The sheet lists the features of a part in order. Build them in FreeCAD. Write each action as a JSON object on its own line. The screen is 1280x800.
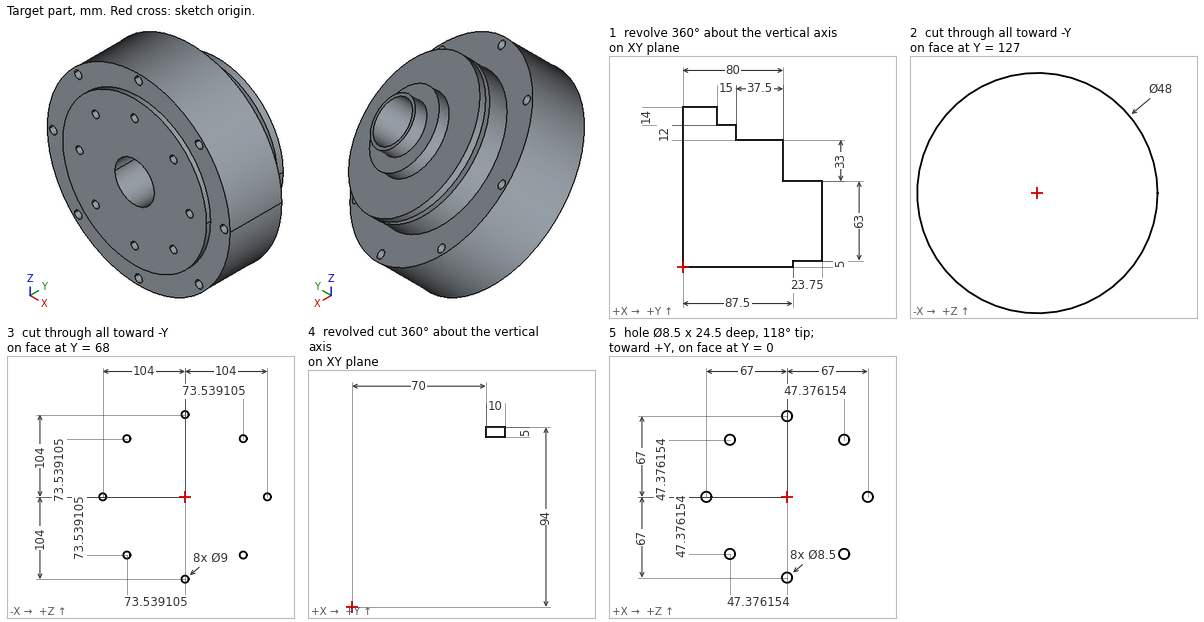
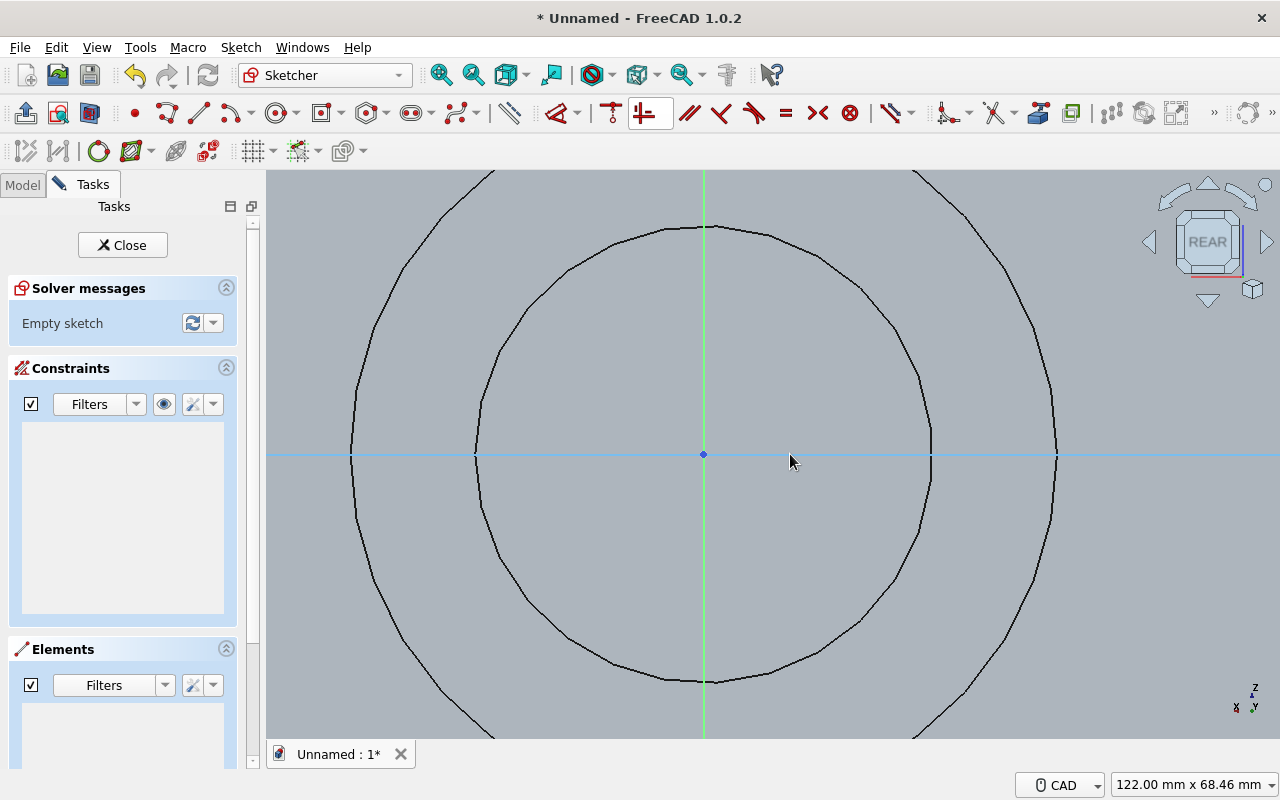
{"action": "left_click", "coordinate": [276, 114]}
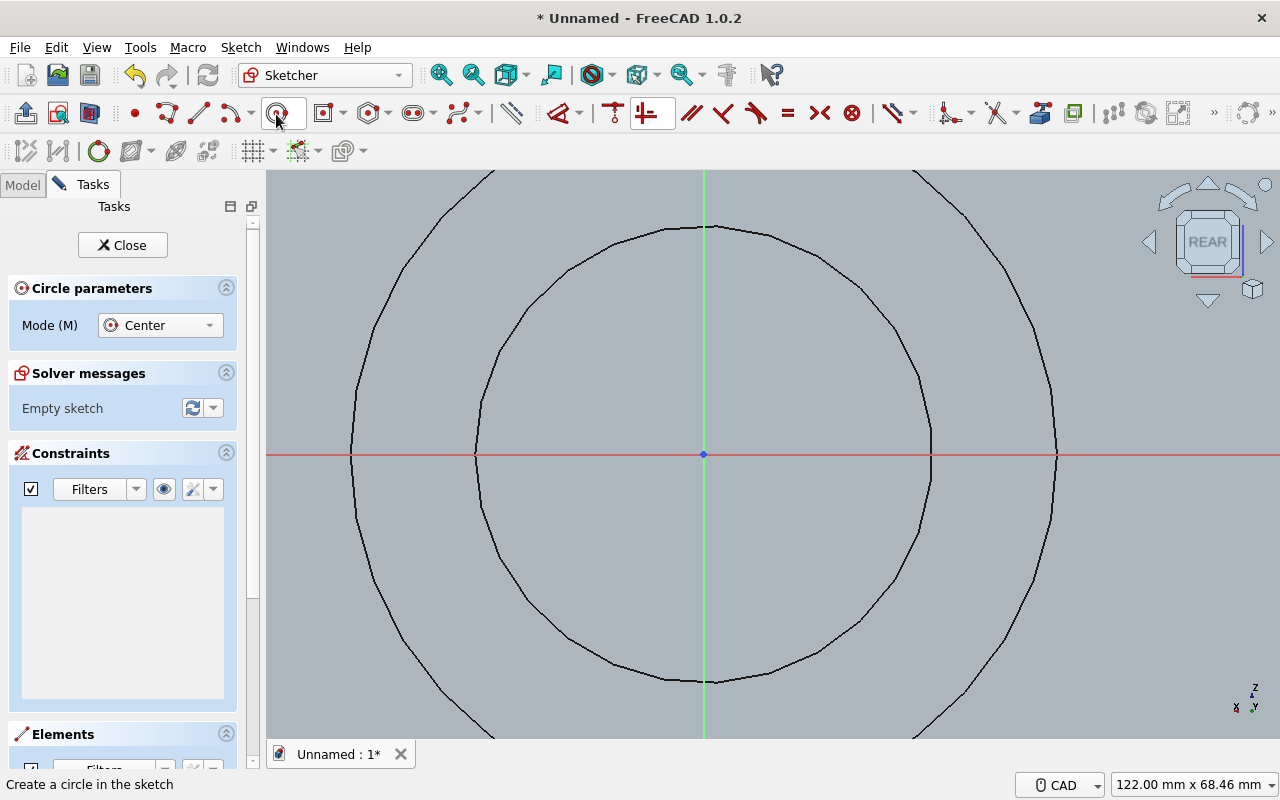
{"action": "left_click", "coordinate": [704, 454]}
{"action": "left_click", "coordinate": [845, 313]}
{"action": "key", "text": "Escape"}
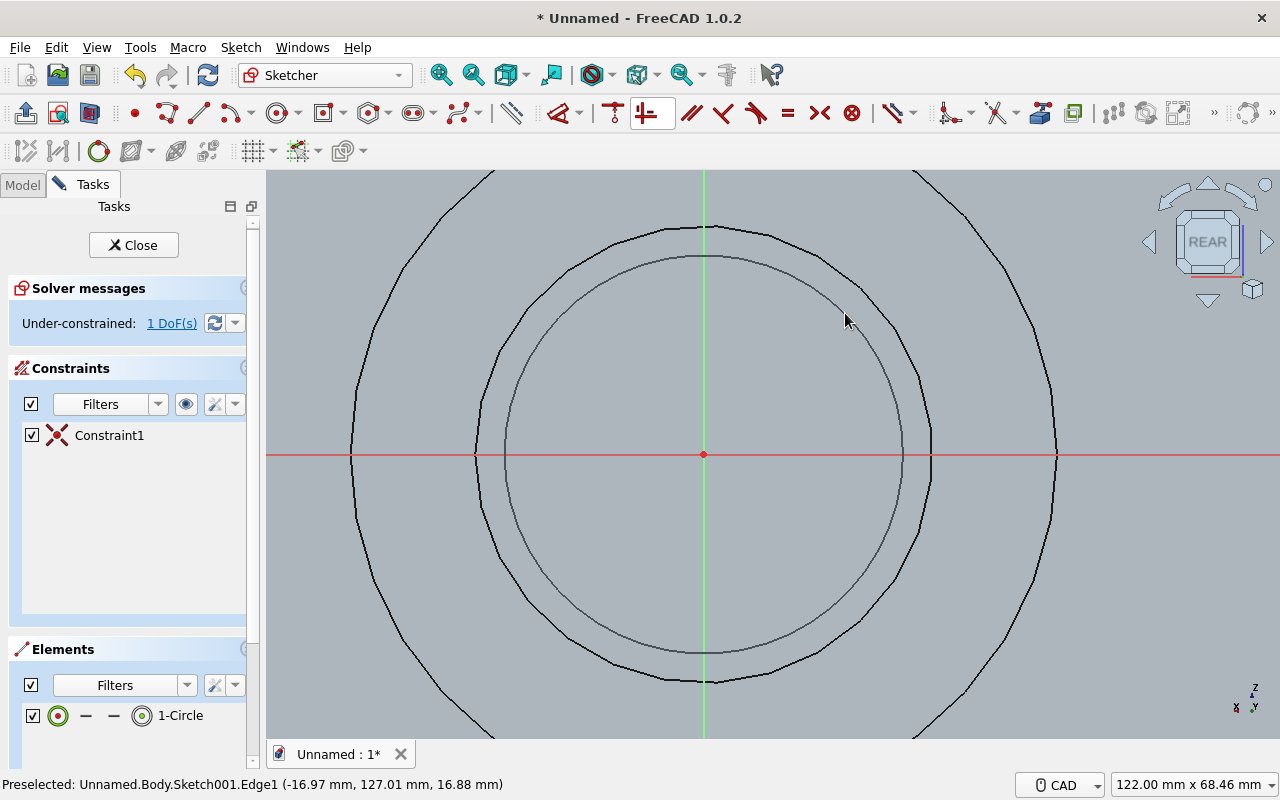
{"action": "left_click", "coordinate": [558, 114]}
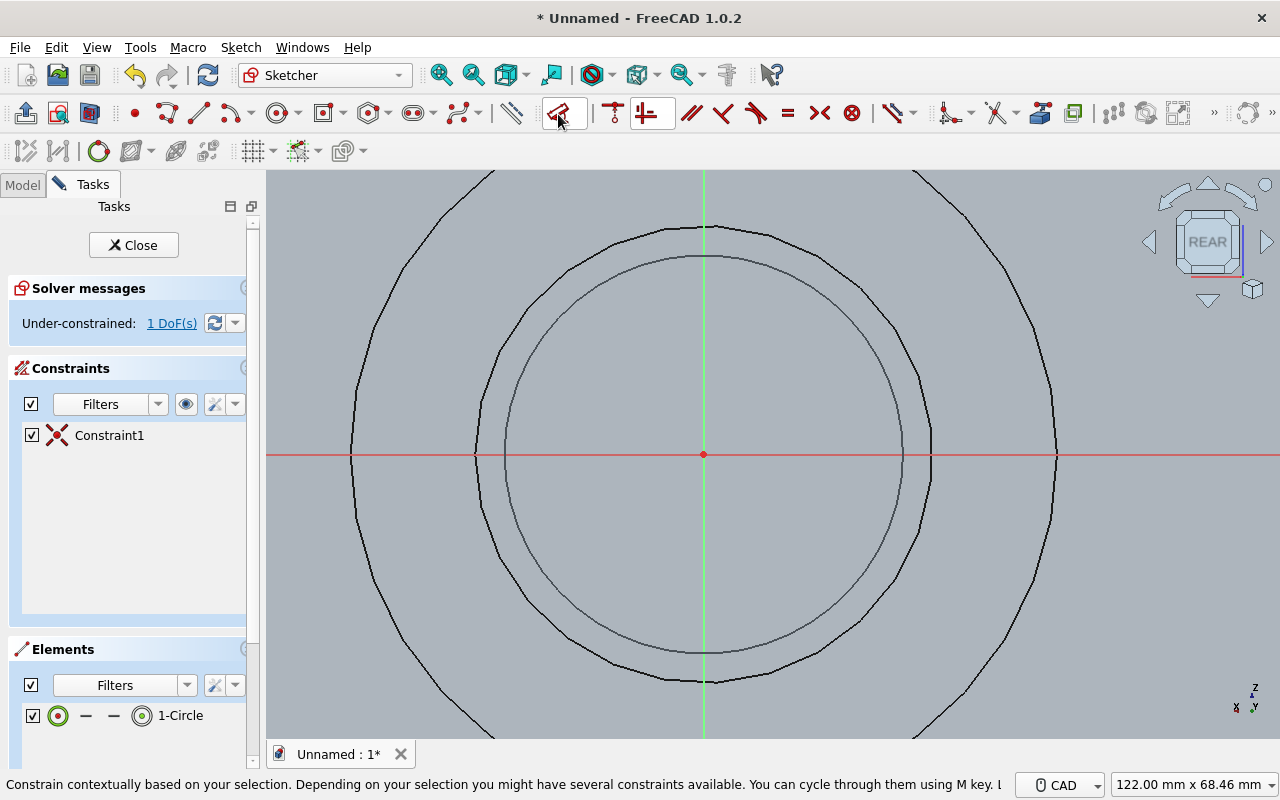
{"action": "left_click", "coordinate": [844, 313]}
{"action": "left_click", "coordinate": [867, 290]}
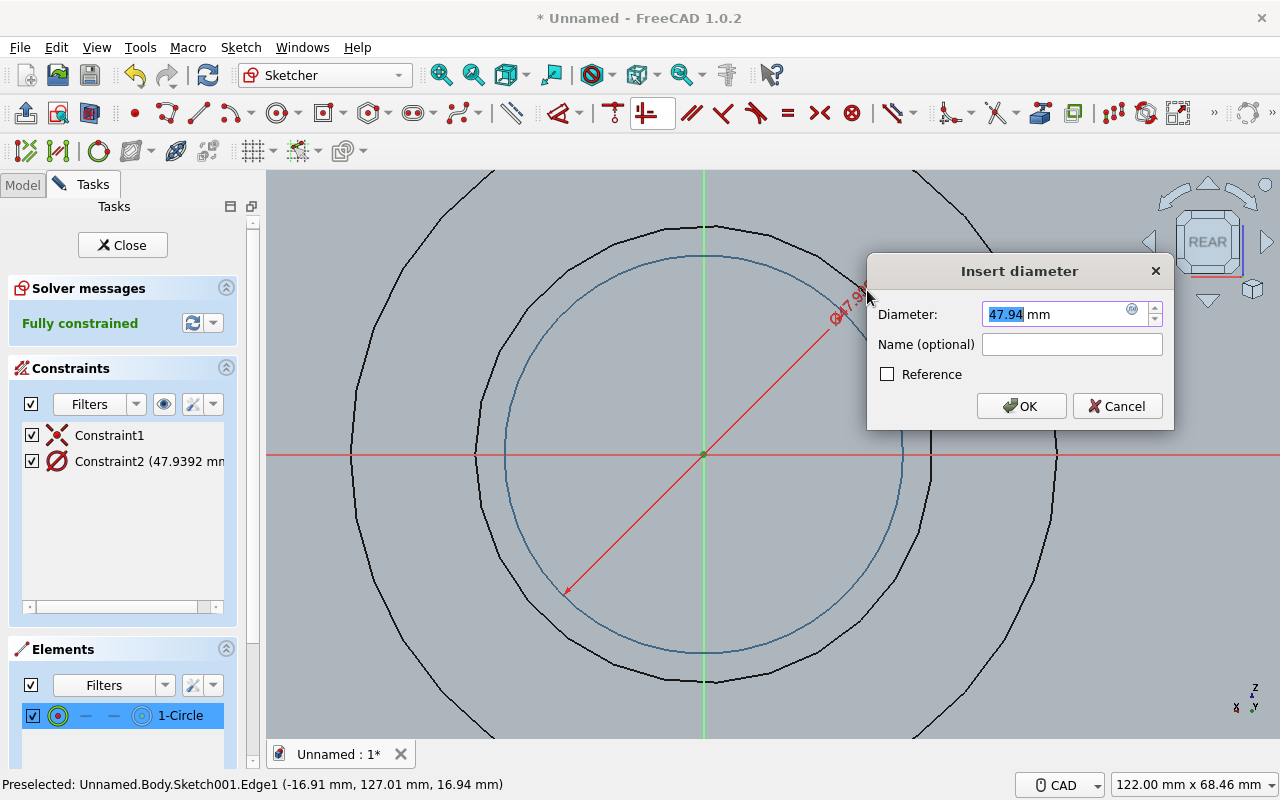
{"action": "type", "text": "48"}
{"action": "key", "text": "Return"}
{"action": "key", "text": "Escape"}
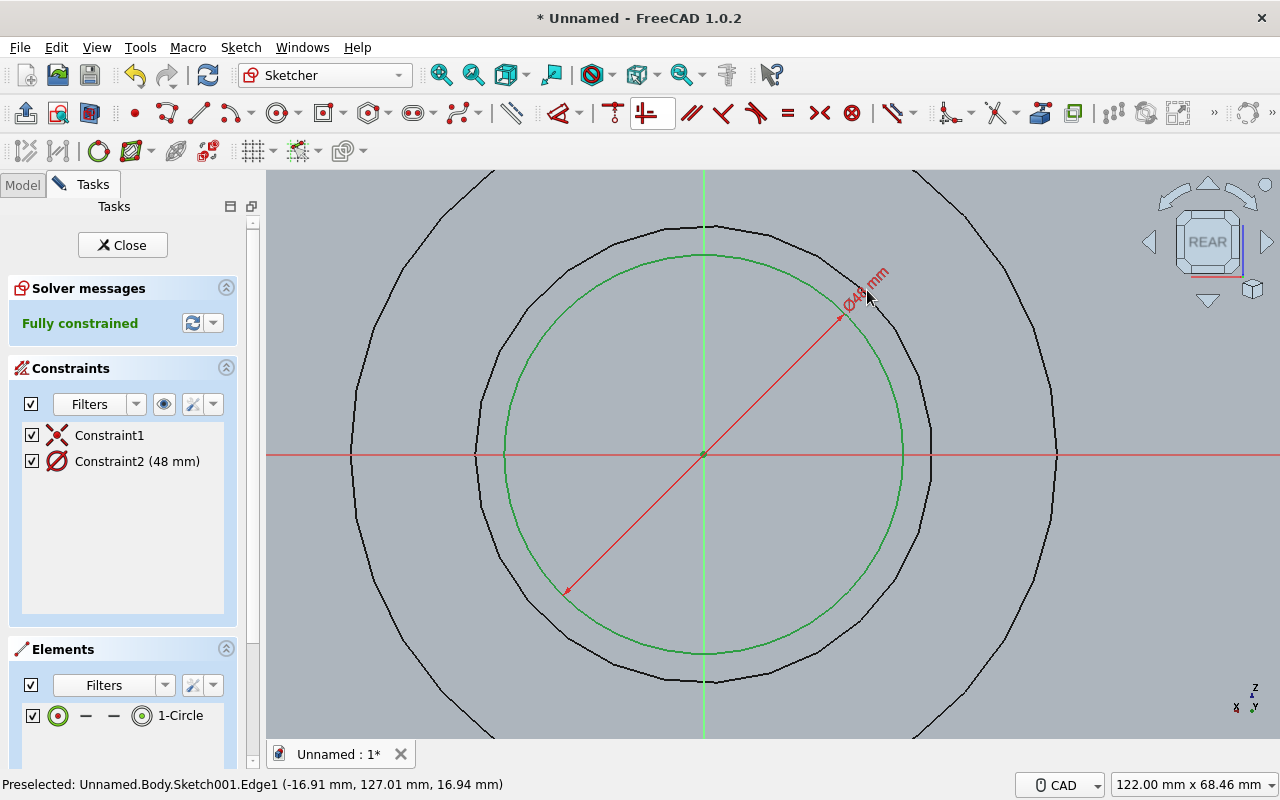
{"action": "left_click", "coordinate": [123, 245]}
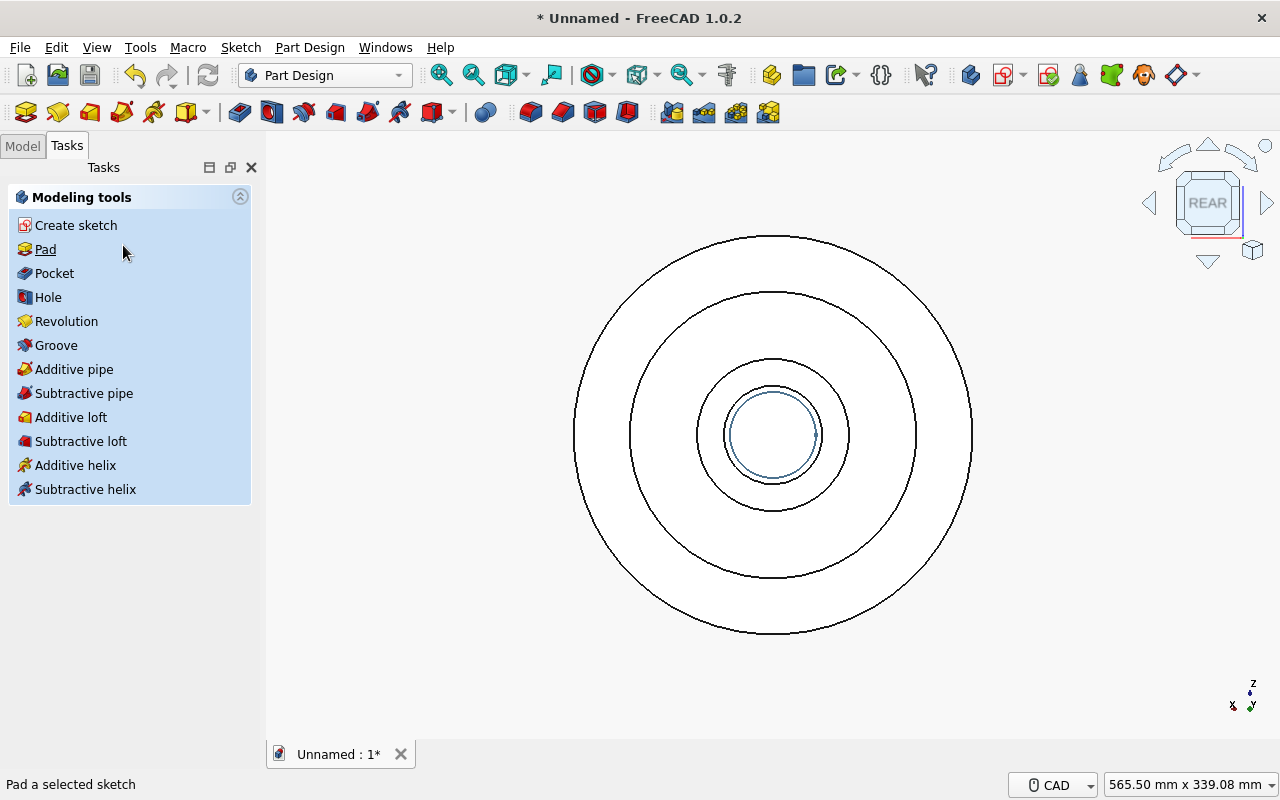
{"action": "left_click", "coordinate": [240, 112]}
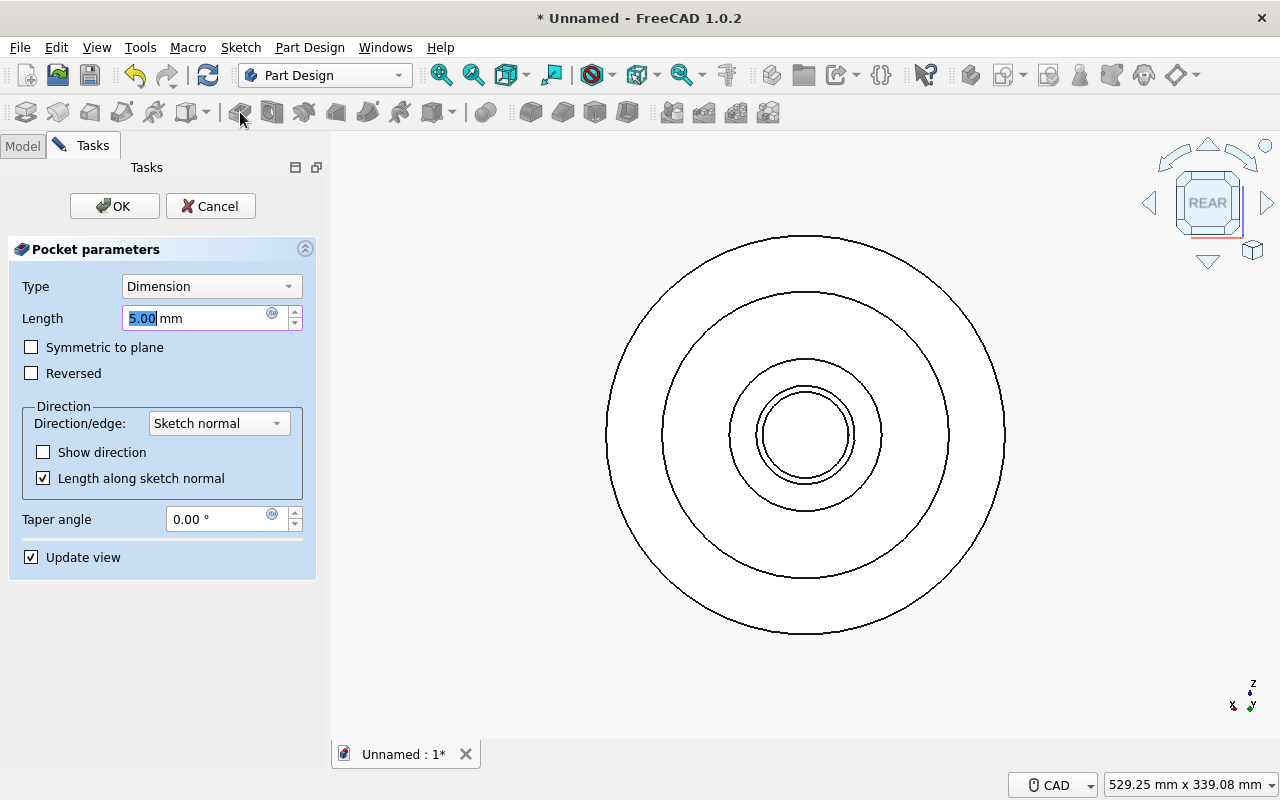
{"action": "left_click", "coordinate": [212, 286]}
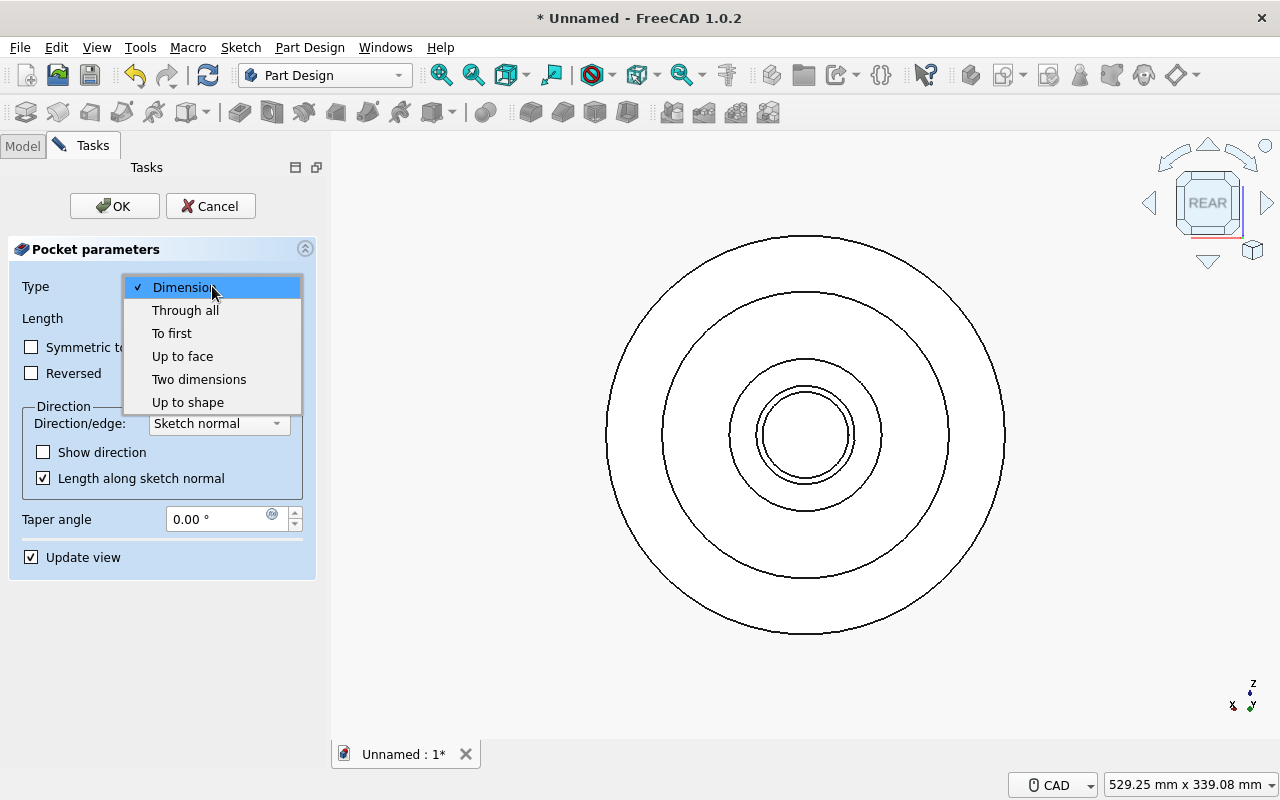
{"action": "left_click", "coordinate": [212, 310]}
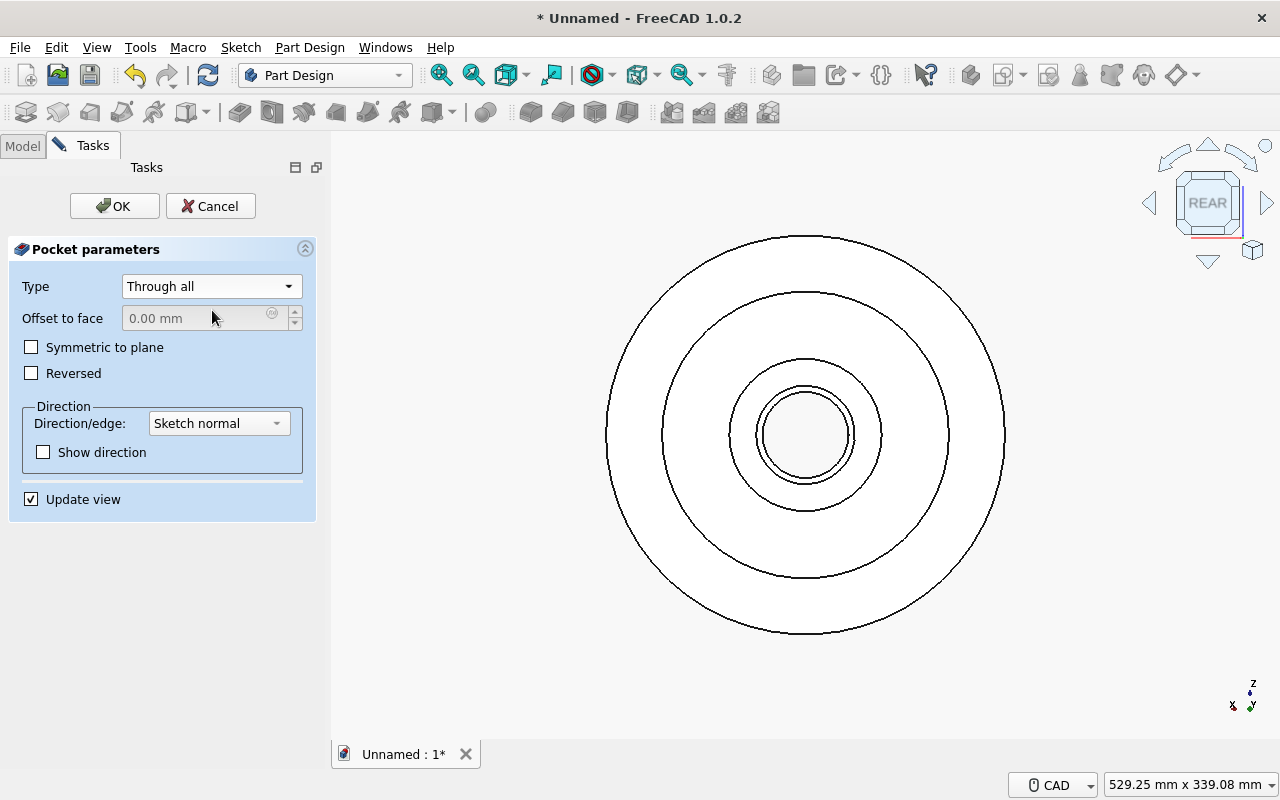
{"action": "left_click", "coordinate": [115, 206]}